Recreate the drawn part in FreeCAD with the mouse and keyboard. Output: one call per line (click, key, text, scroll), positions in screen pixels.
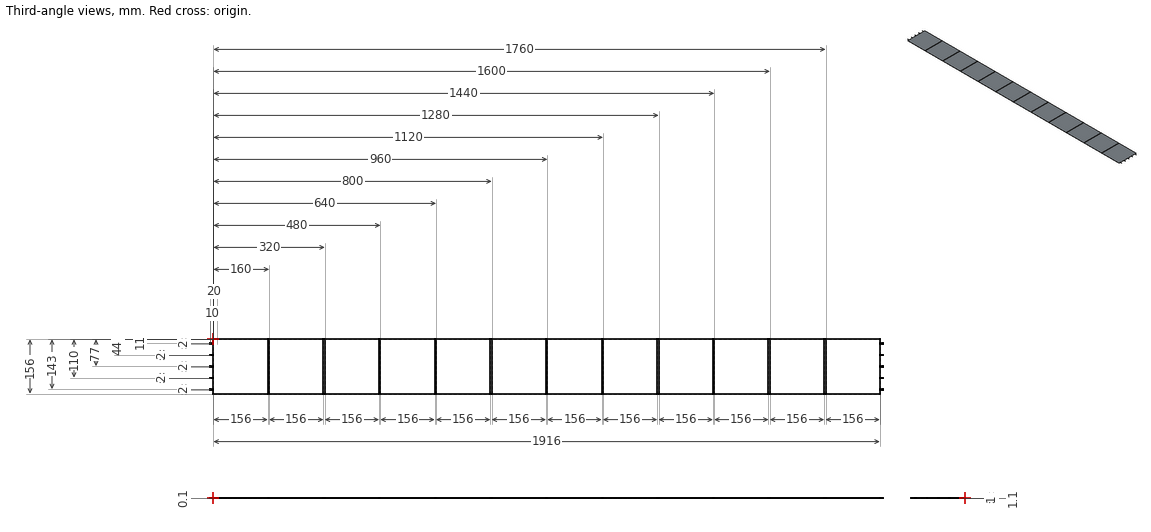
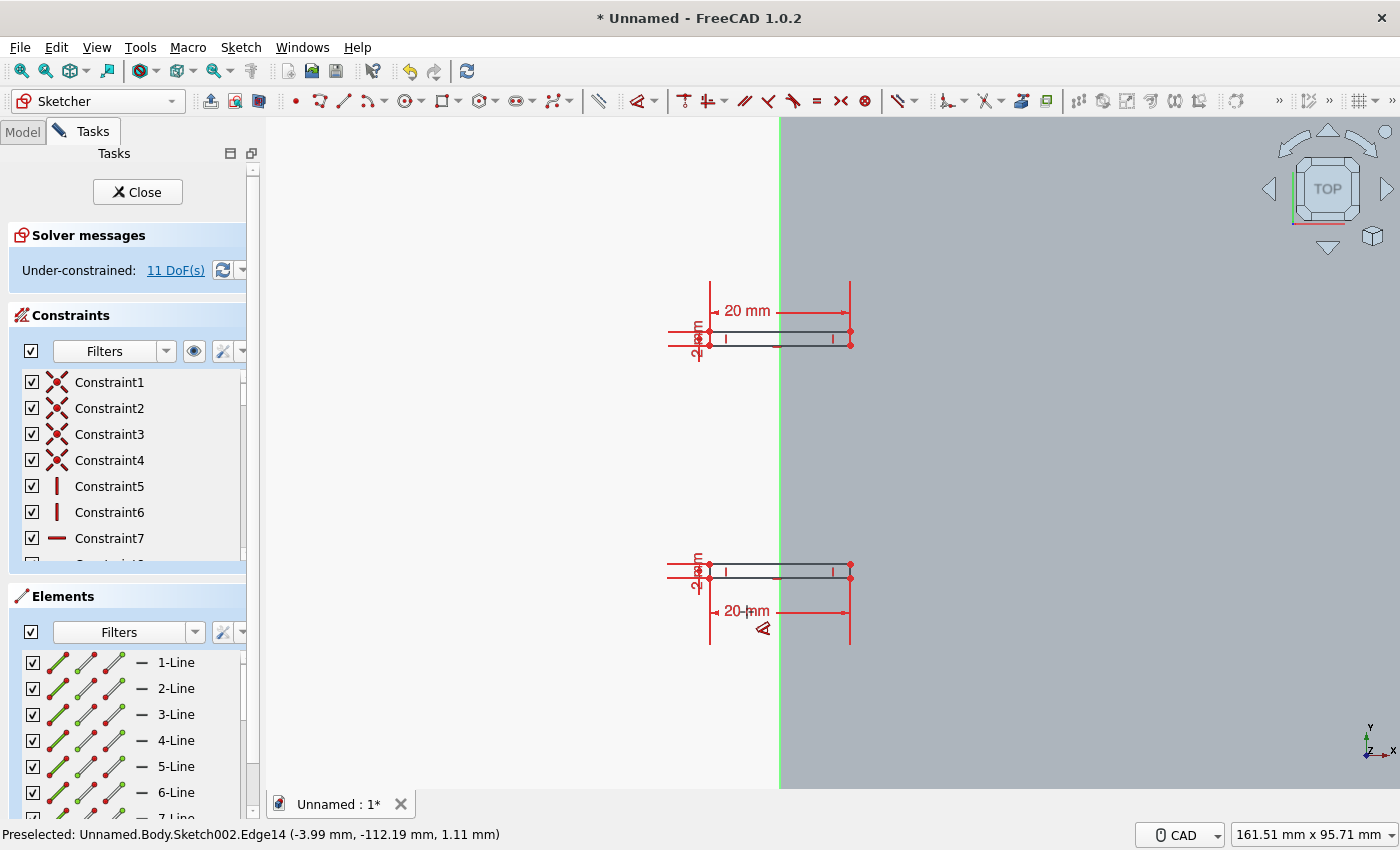
scroll(752, 578, down, 4)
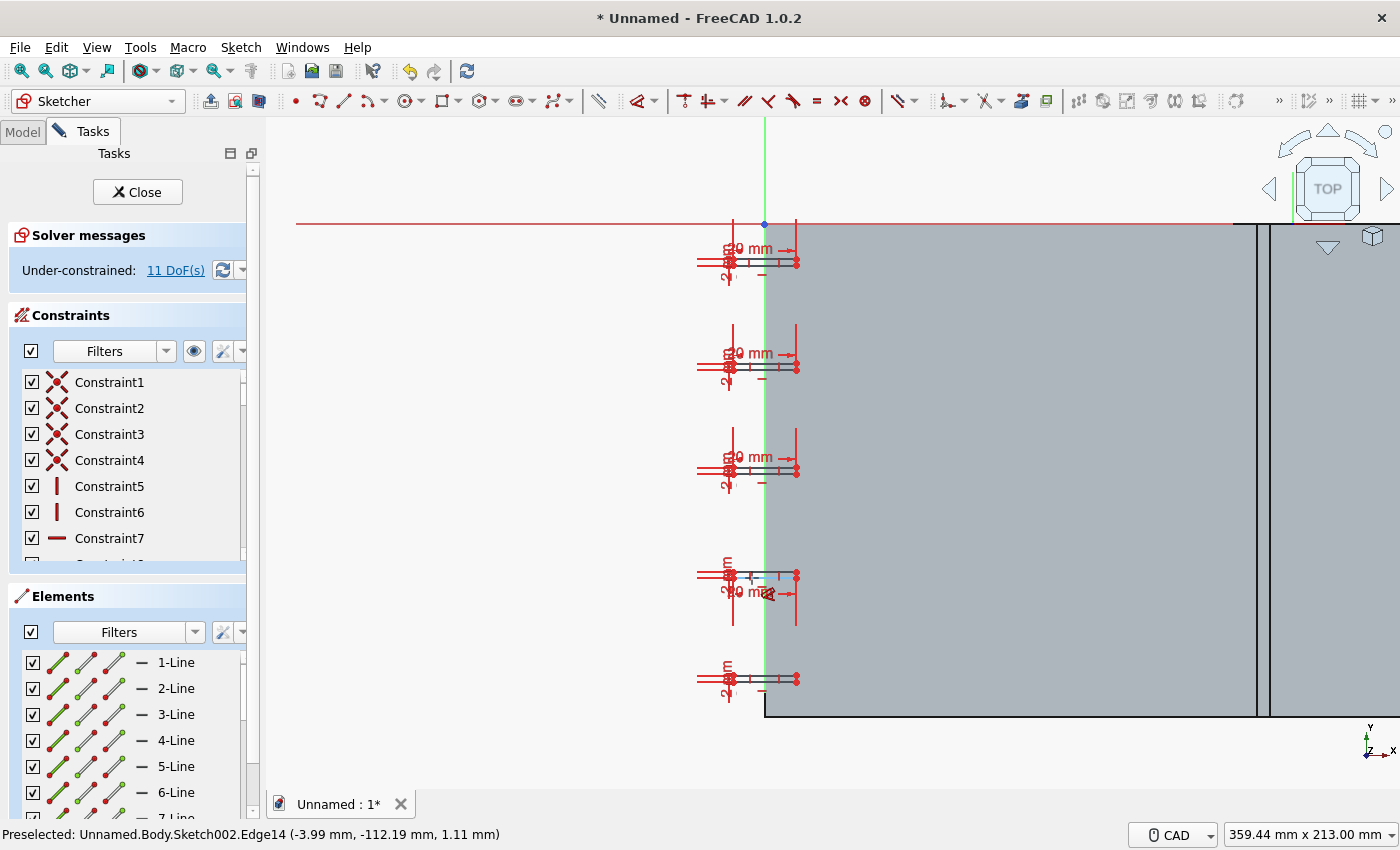
scroll(752, 682, up, 4)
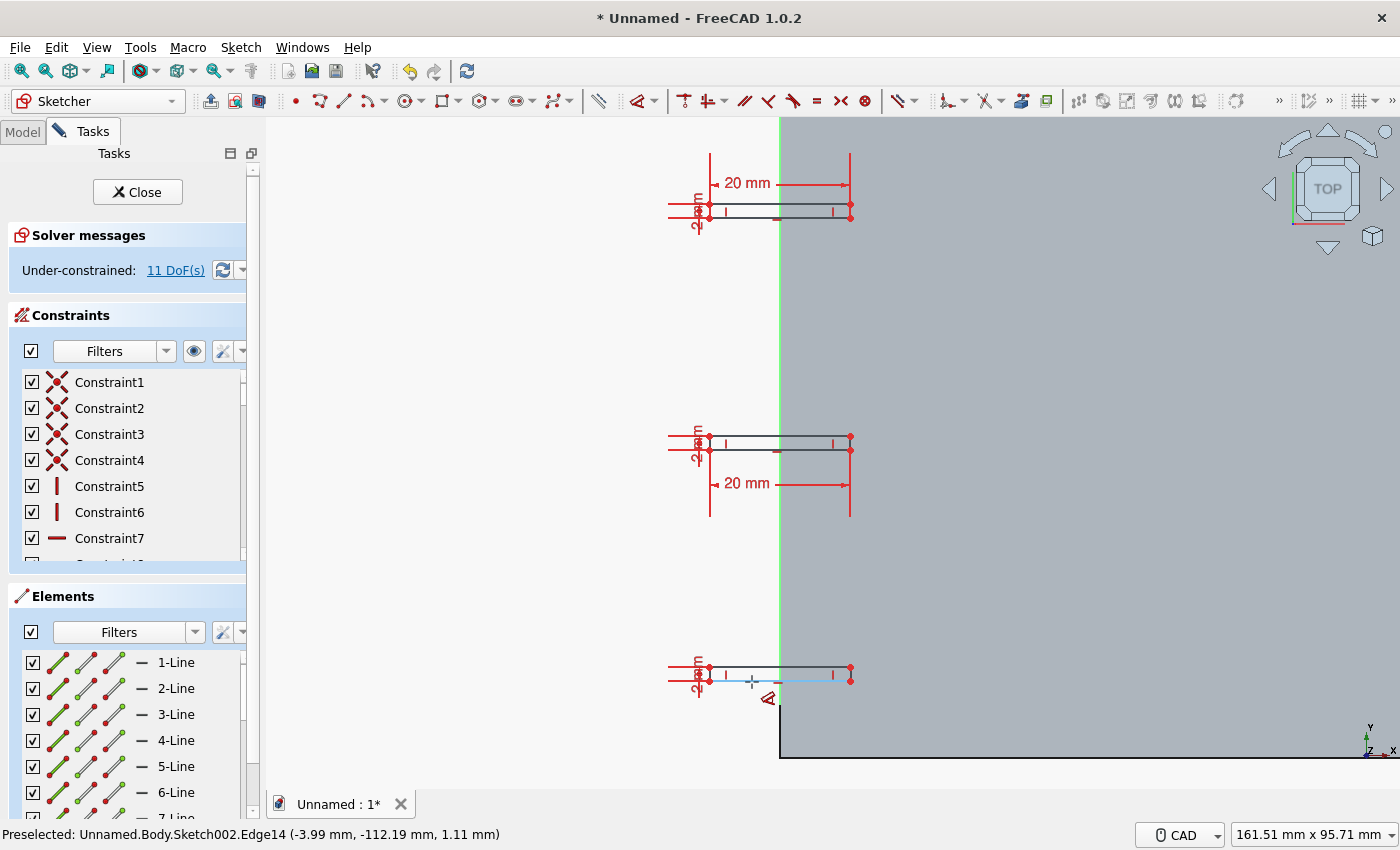
click(752, 681)
click(748, 715)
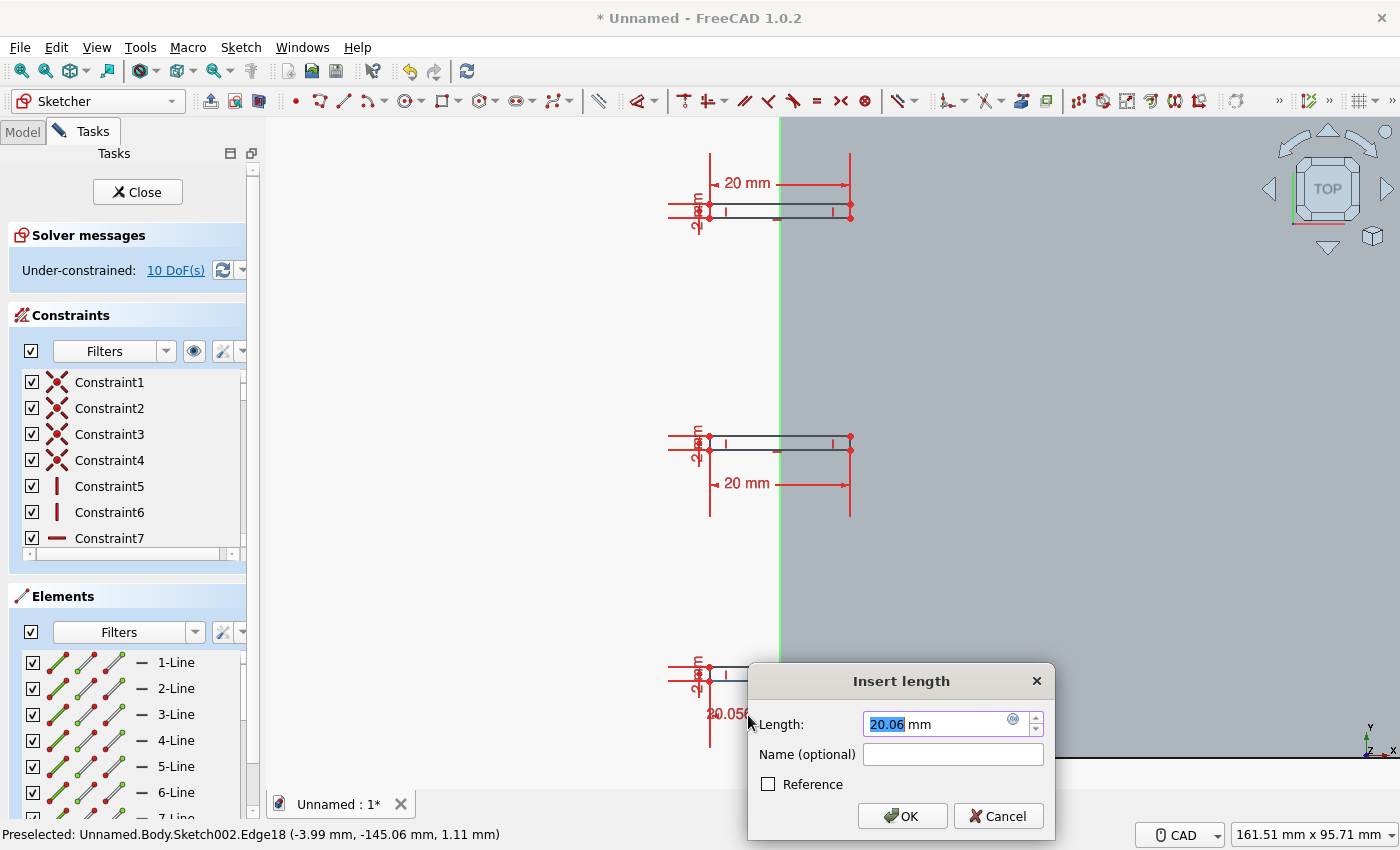
text(20)
key(Return)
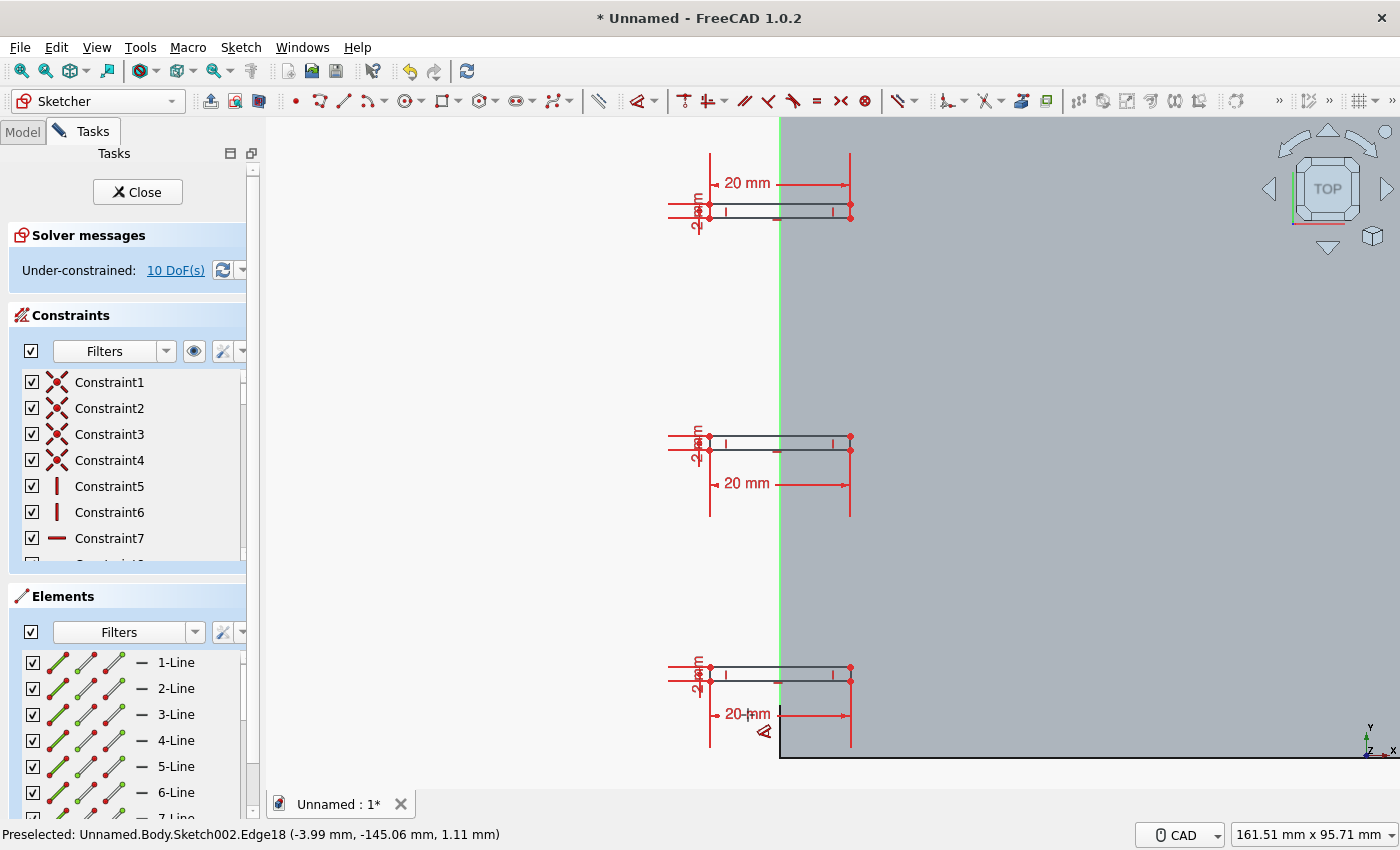
scroll(752, 682, down, 4)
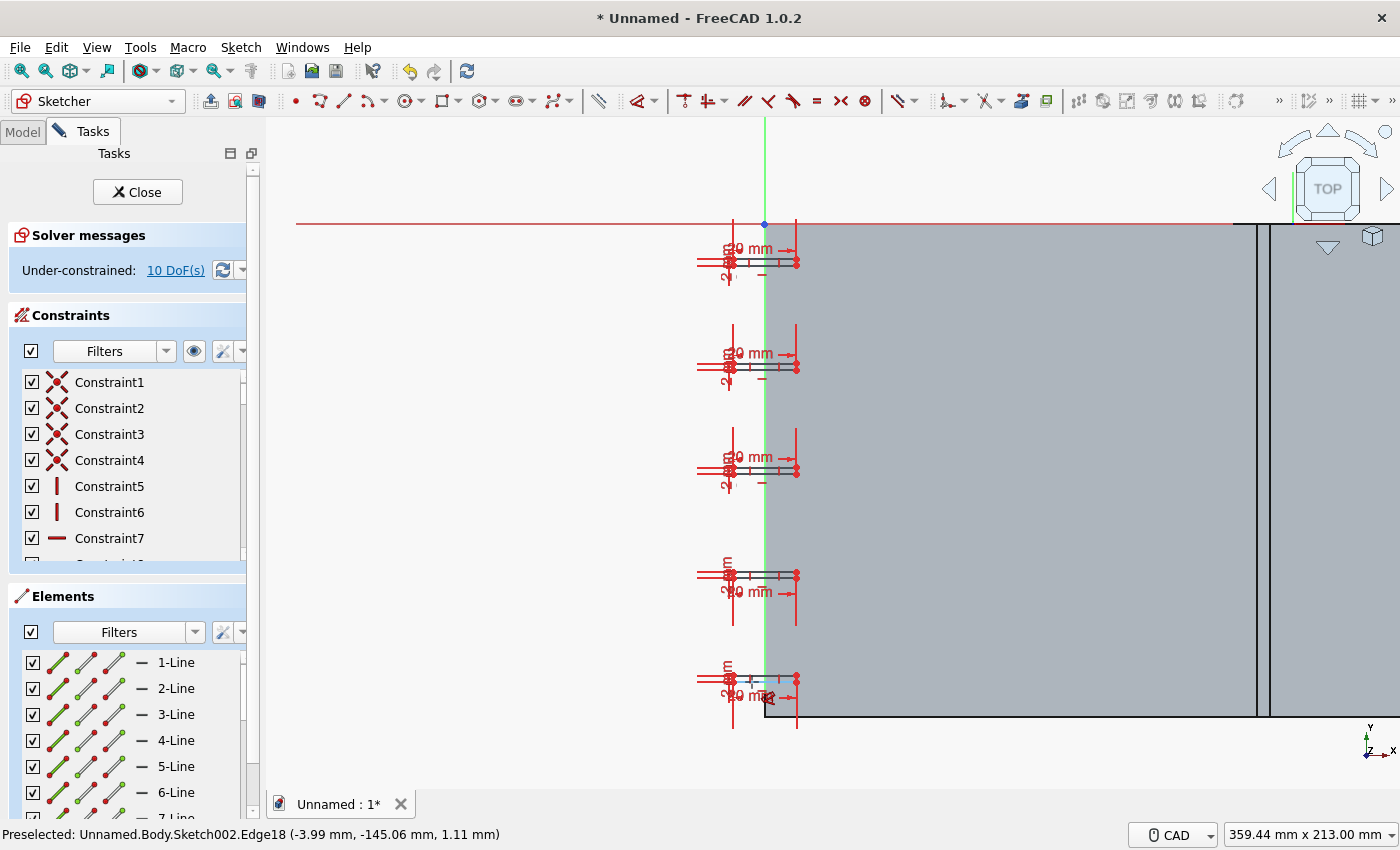
scroll(733, 259, up, 4)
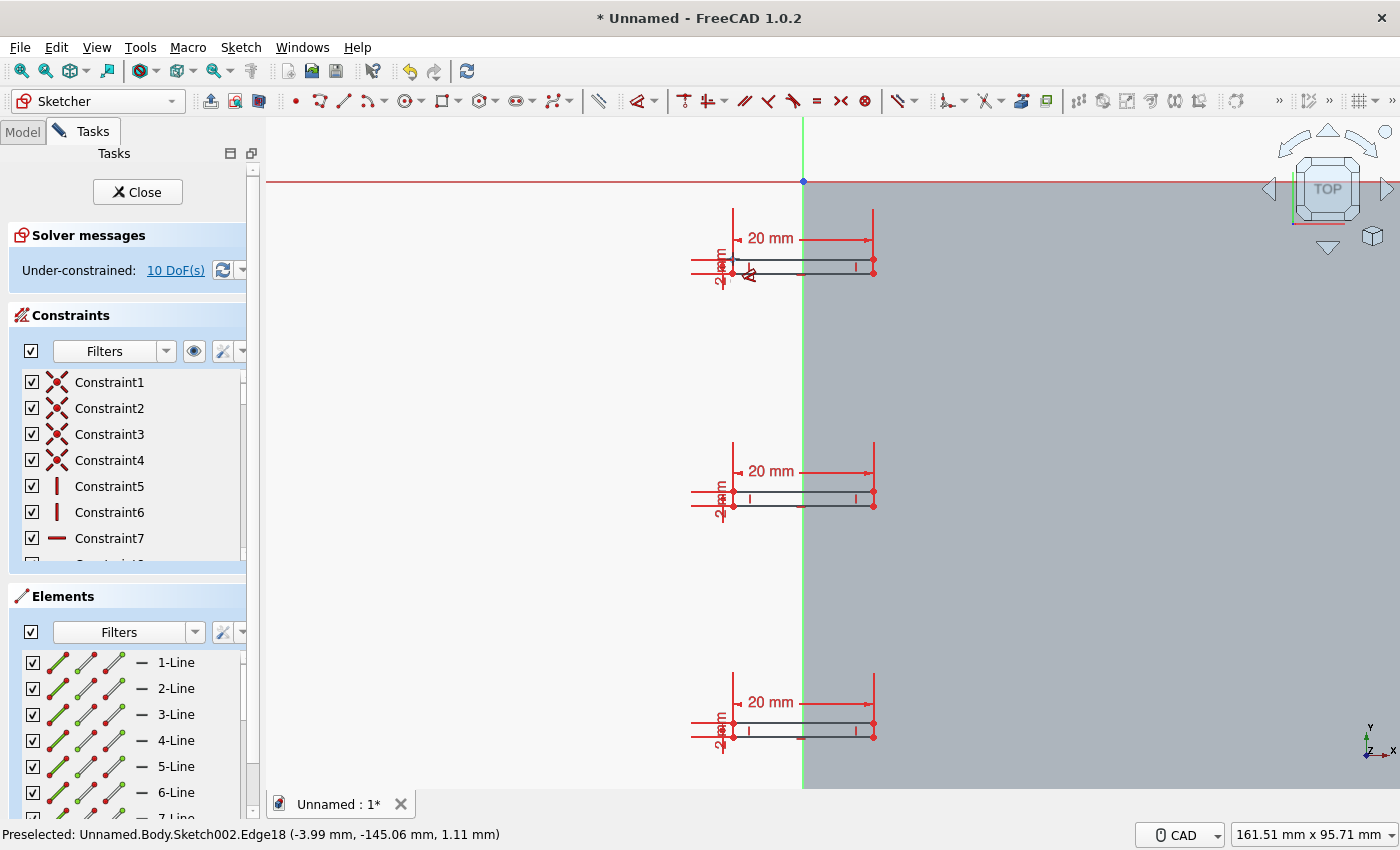
click(733, 260)
click(768, 148)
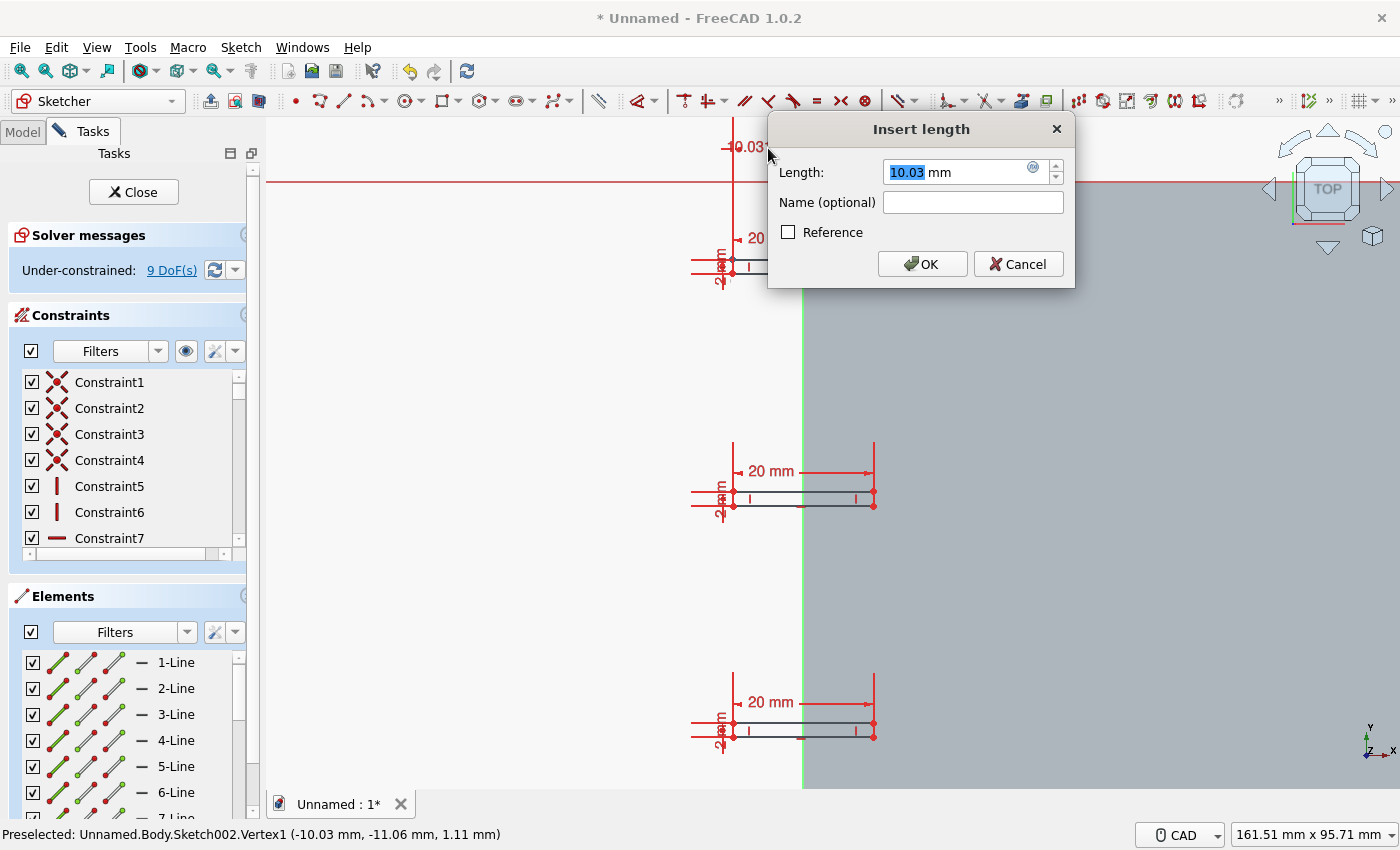
text(10)
key(Return)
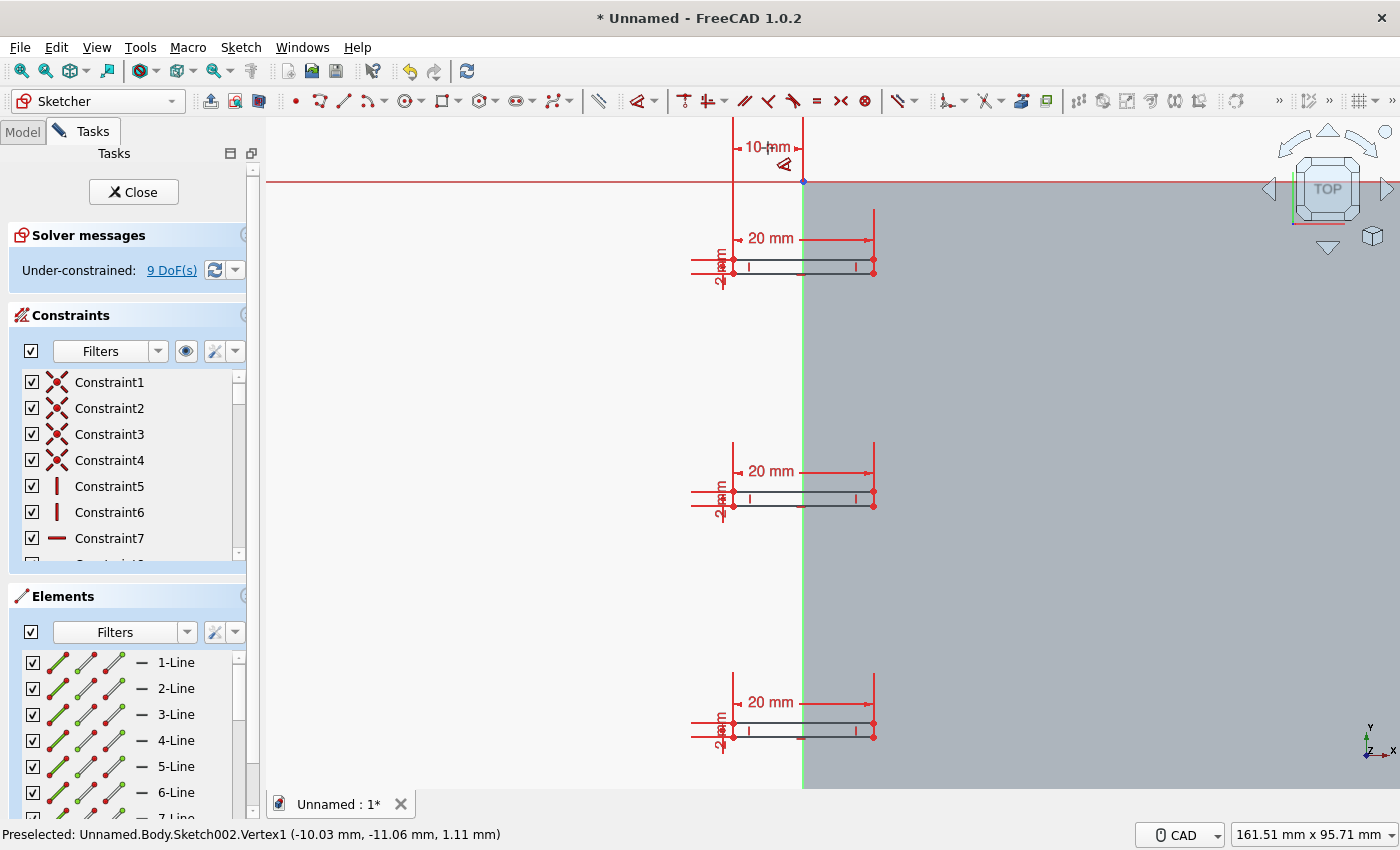
click(733, 260)
click(699, 221)